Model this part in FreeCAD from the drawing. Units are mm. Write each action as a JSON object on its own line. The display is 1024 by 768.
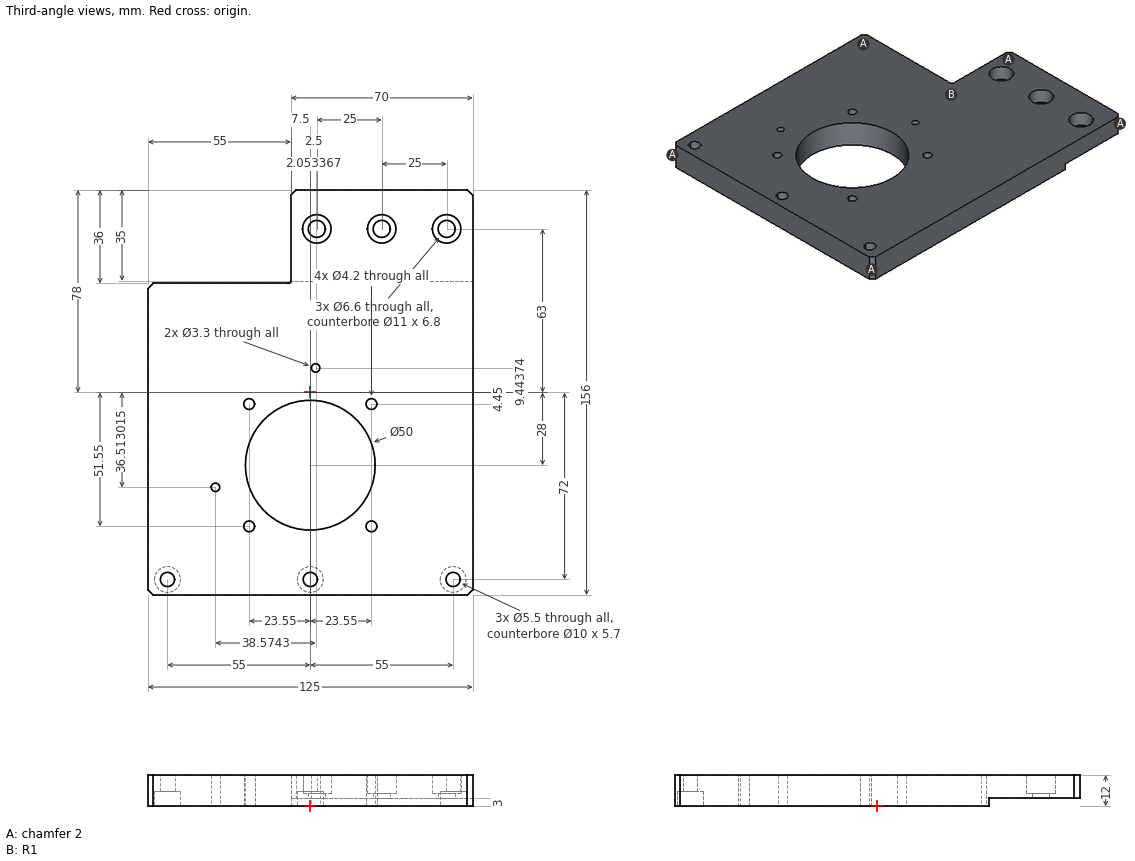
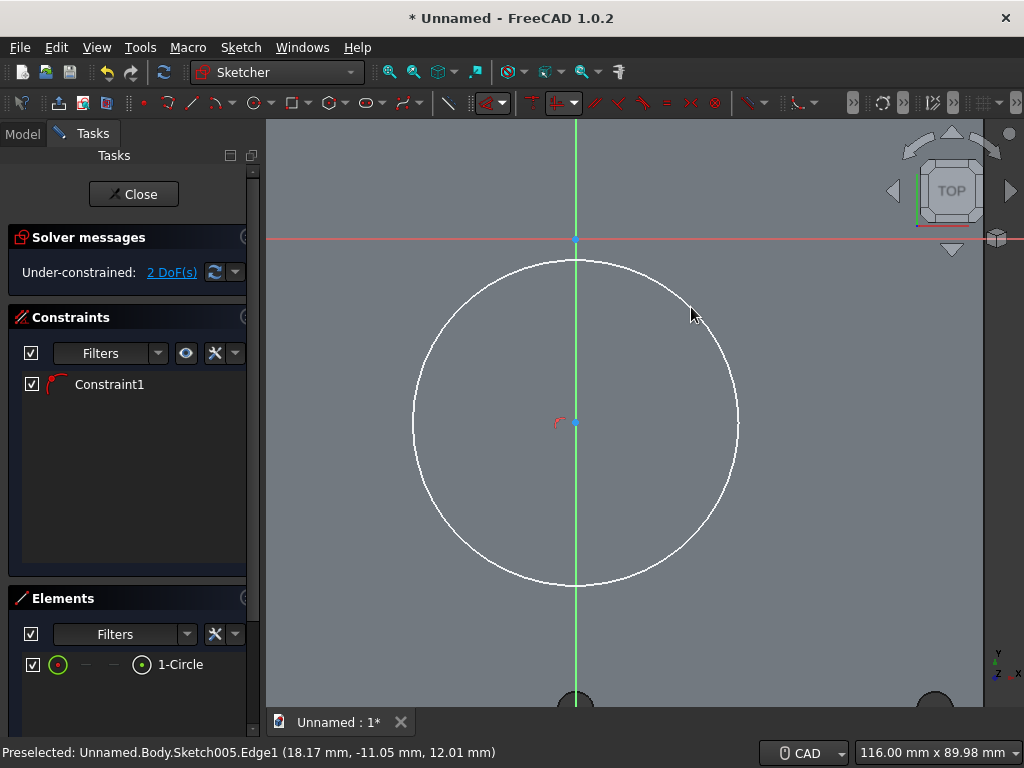
{"action": "left_click", "coordinate": [690, 307]}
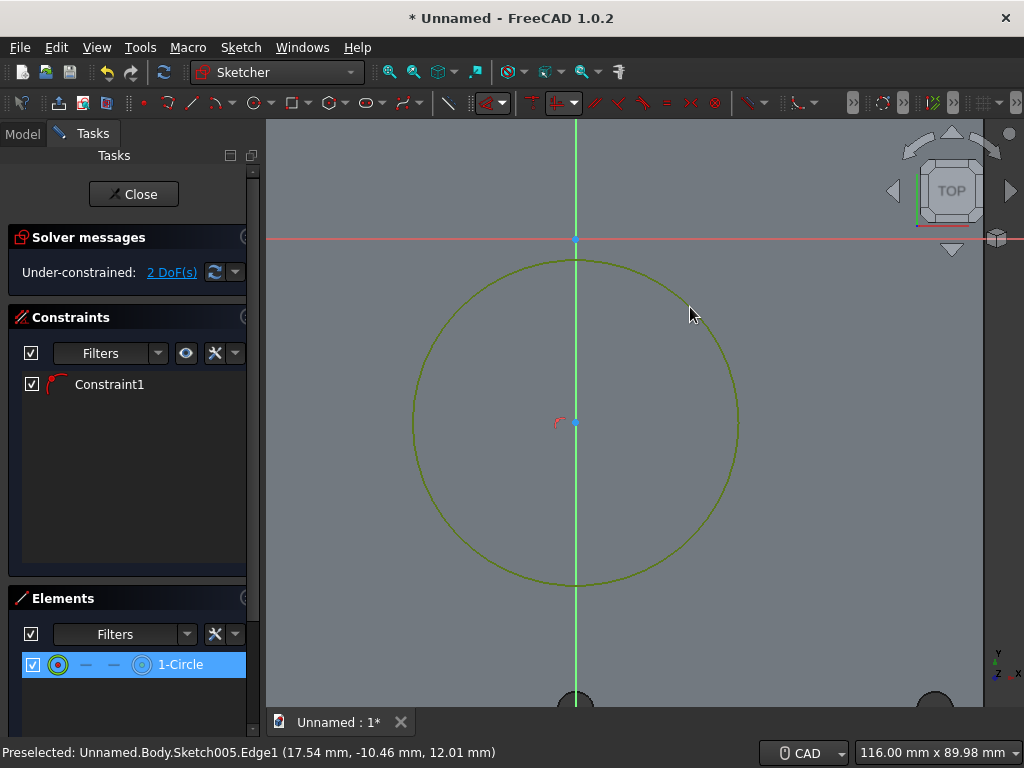
{"action": "left_click", "coordinate": [504, 104]}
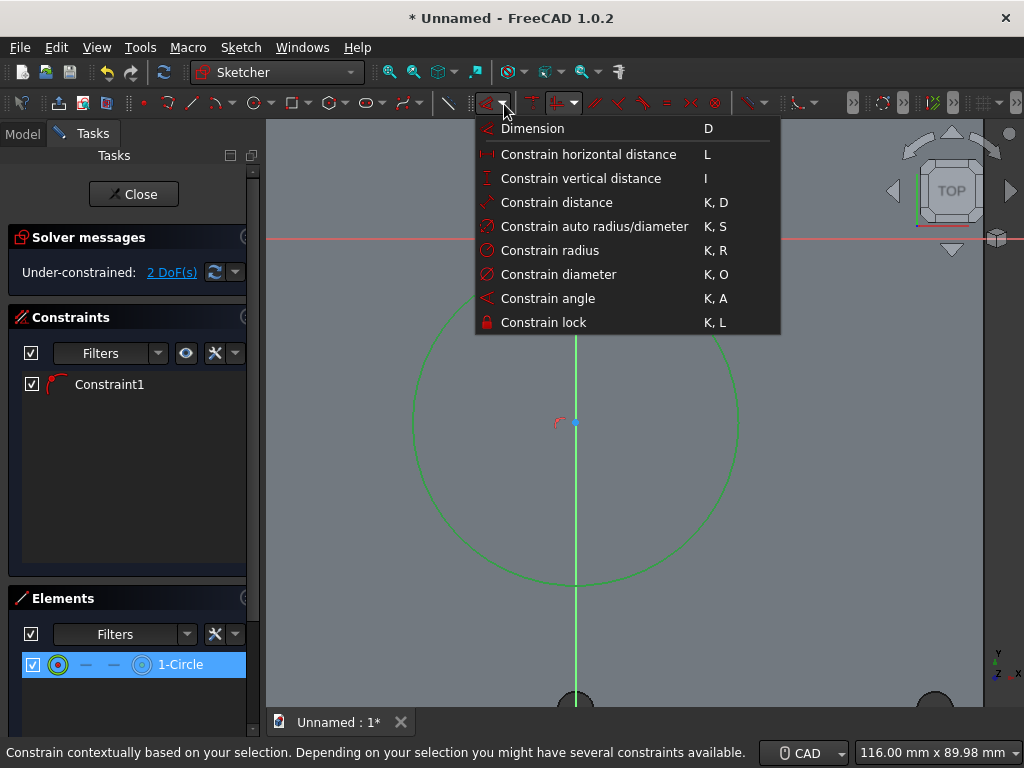
{"action": "left_click", "coordinate": [628, 274]}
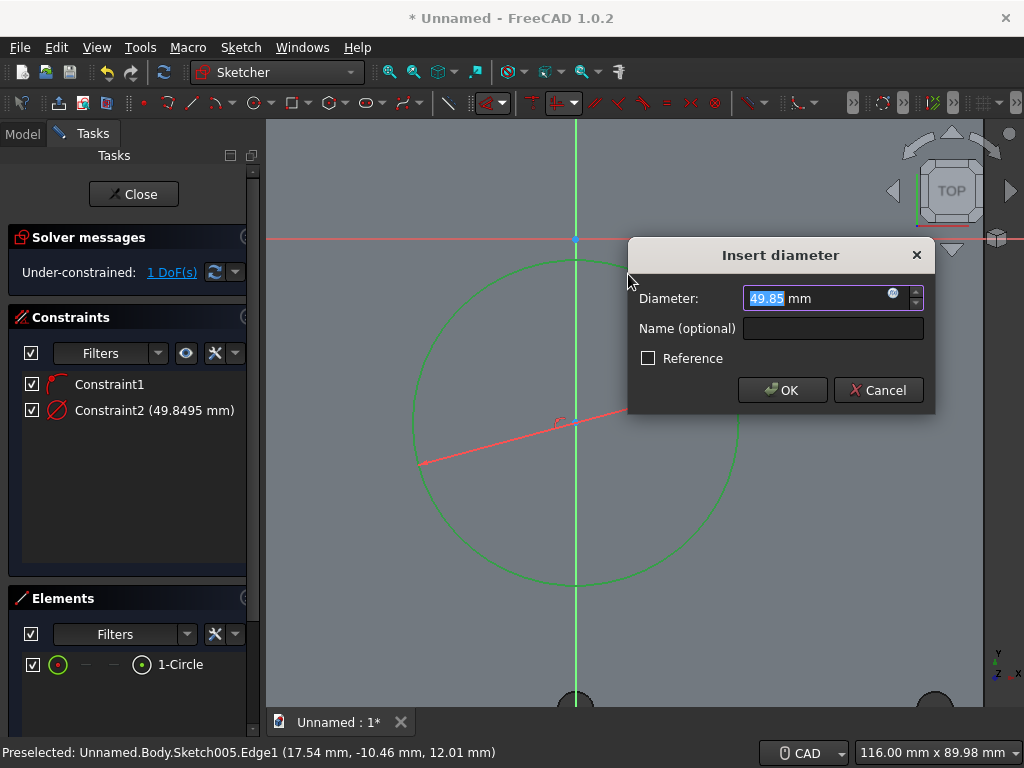
{"action": "type", "text": "50"}
{"action": "key", "text": "Return"}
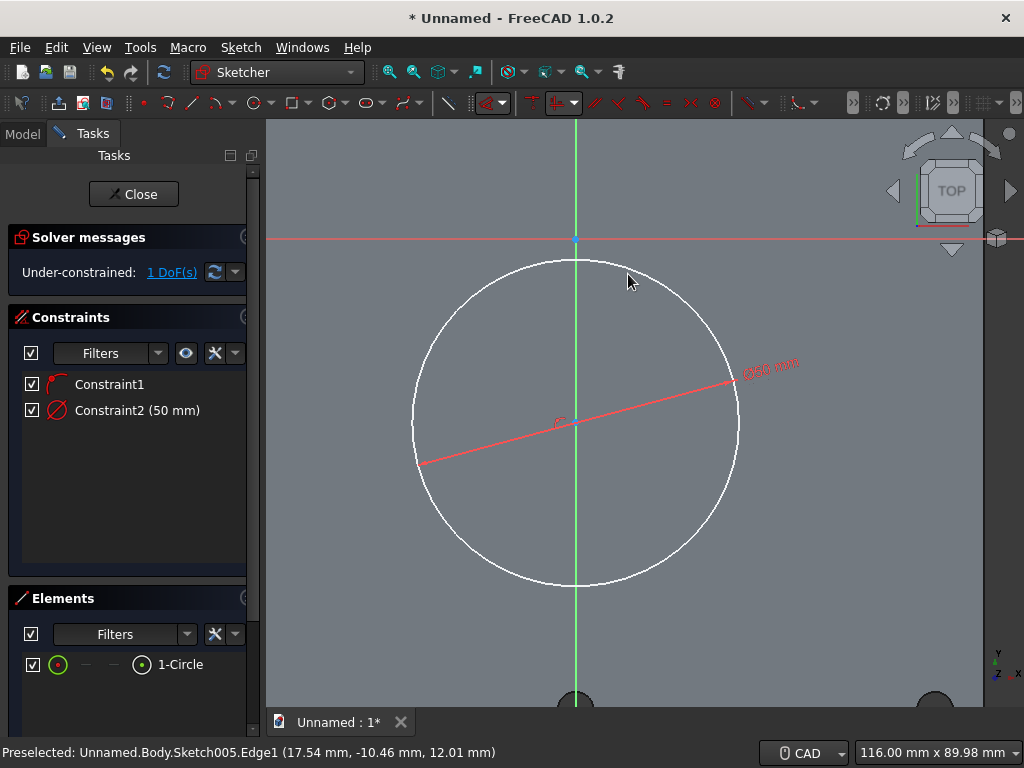
{"action": "left_click", "coordinate": [576, 423]}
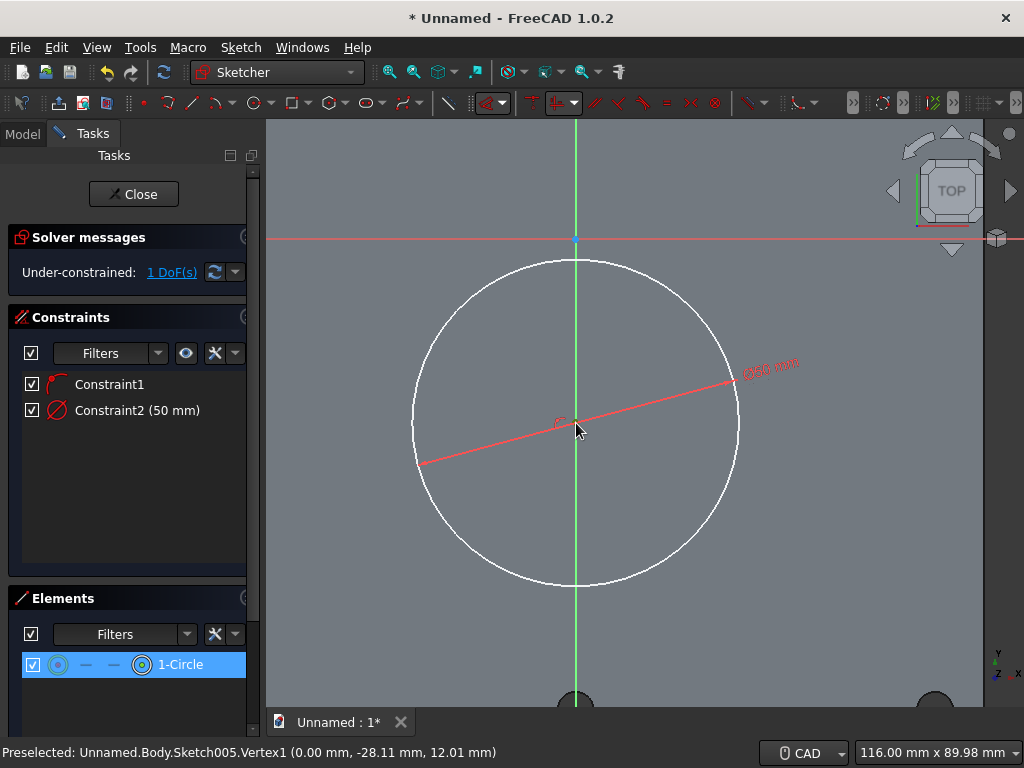
{"action": "left_click", "coordinate": [504, 104]}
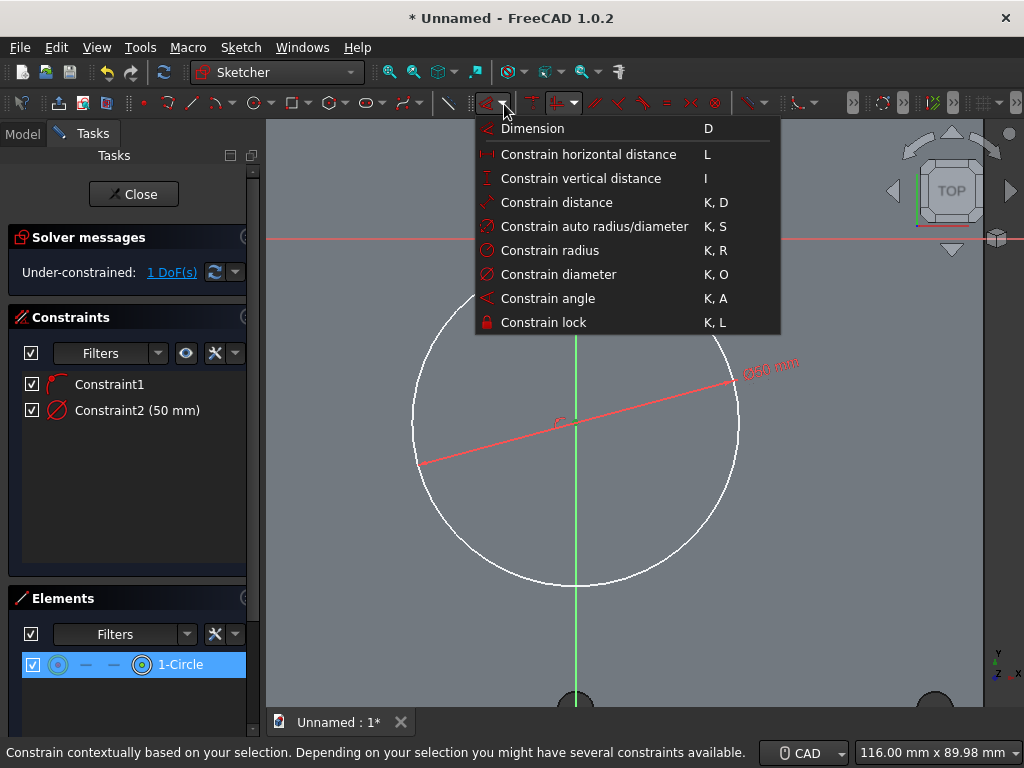
{"action": "left_click", "coordinate": [628, 178]}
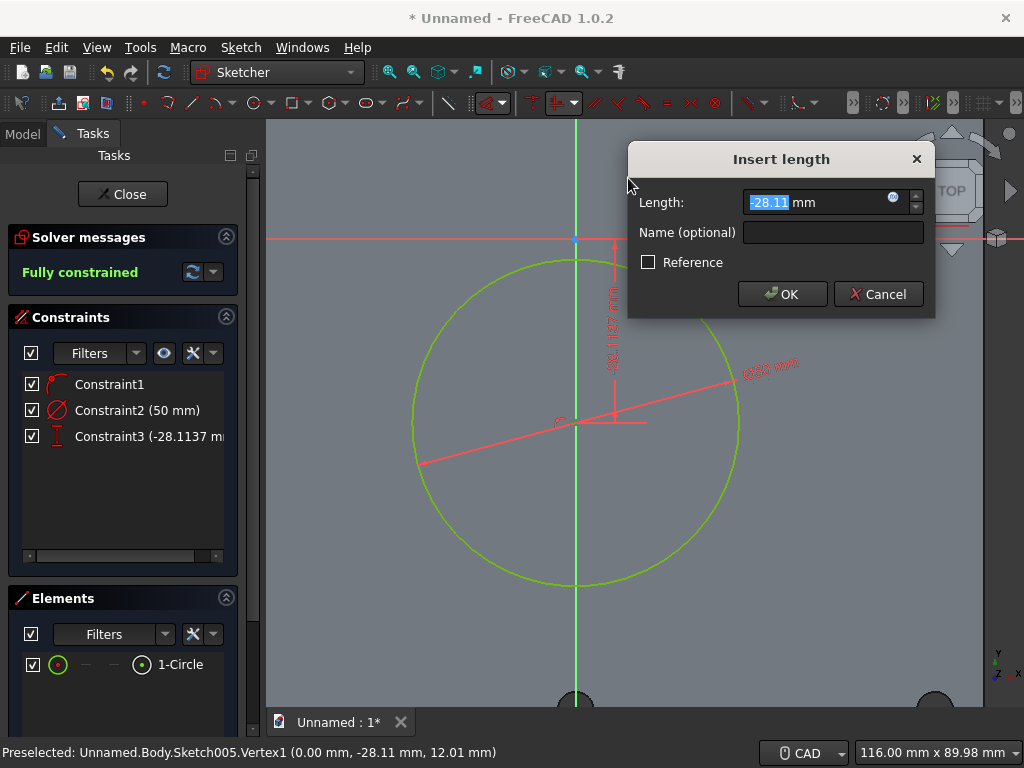
{"action": "type", "text": "-28"}
{"action": "key", "text": "Return"}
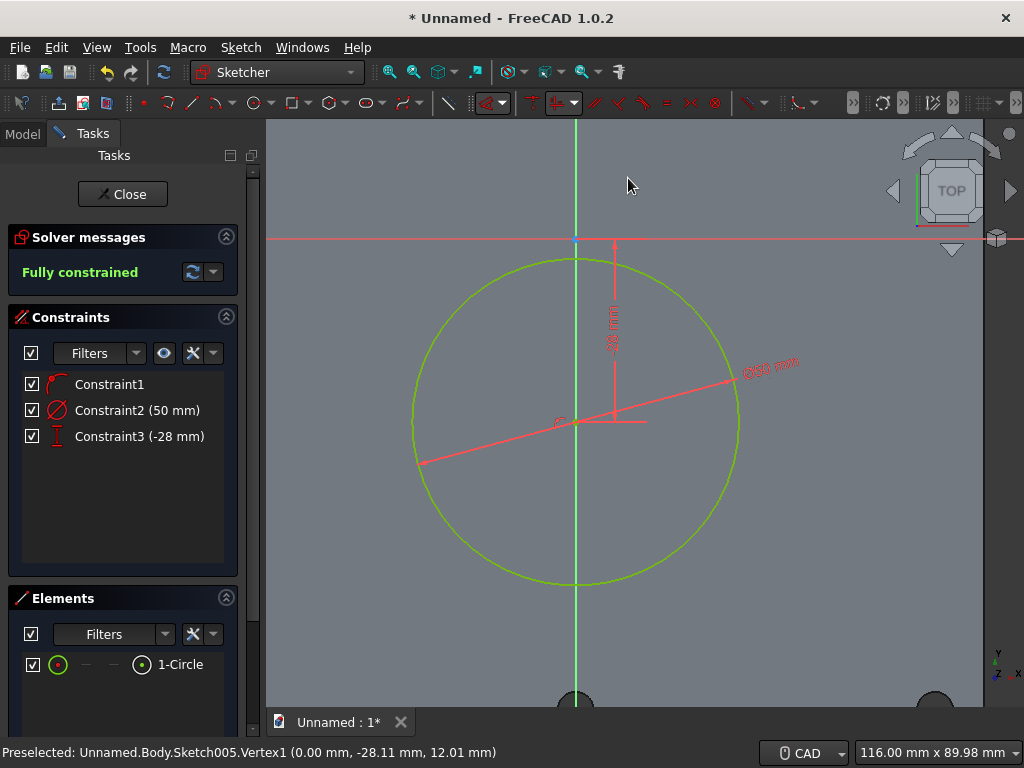
{"action": "left_click", "coordinate": [123, 194]}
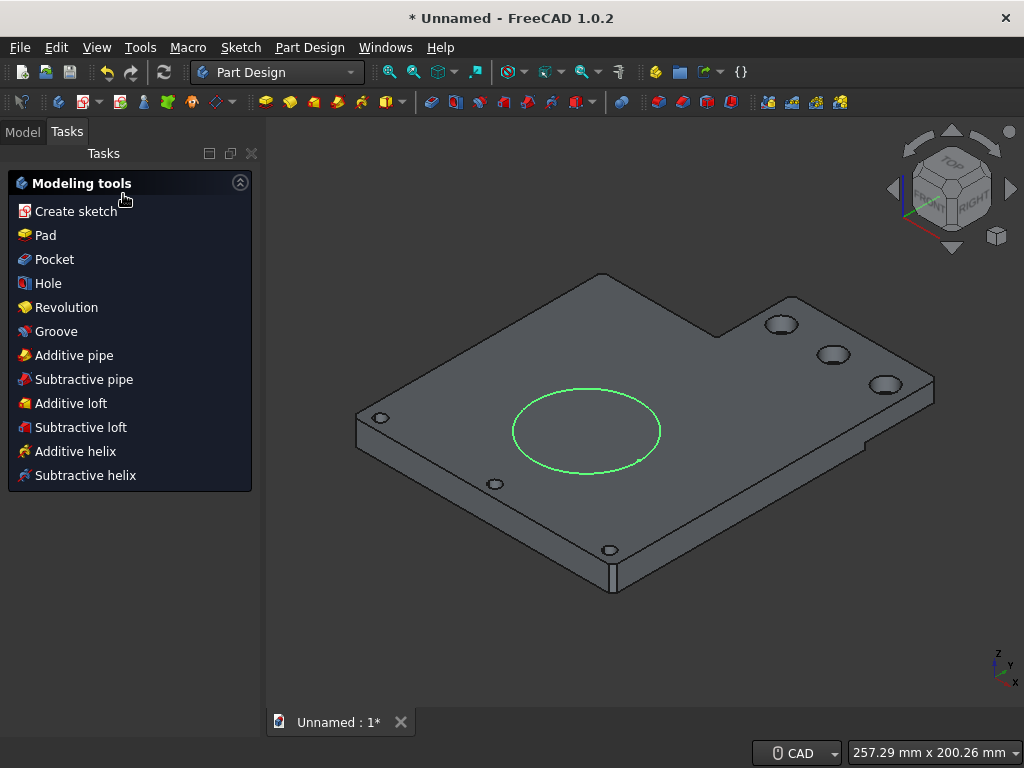
{"action": "left_click", "coordinate": [432, 102]}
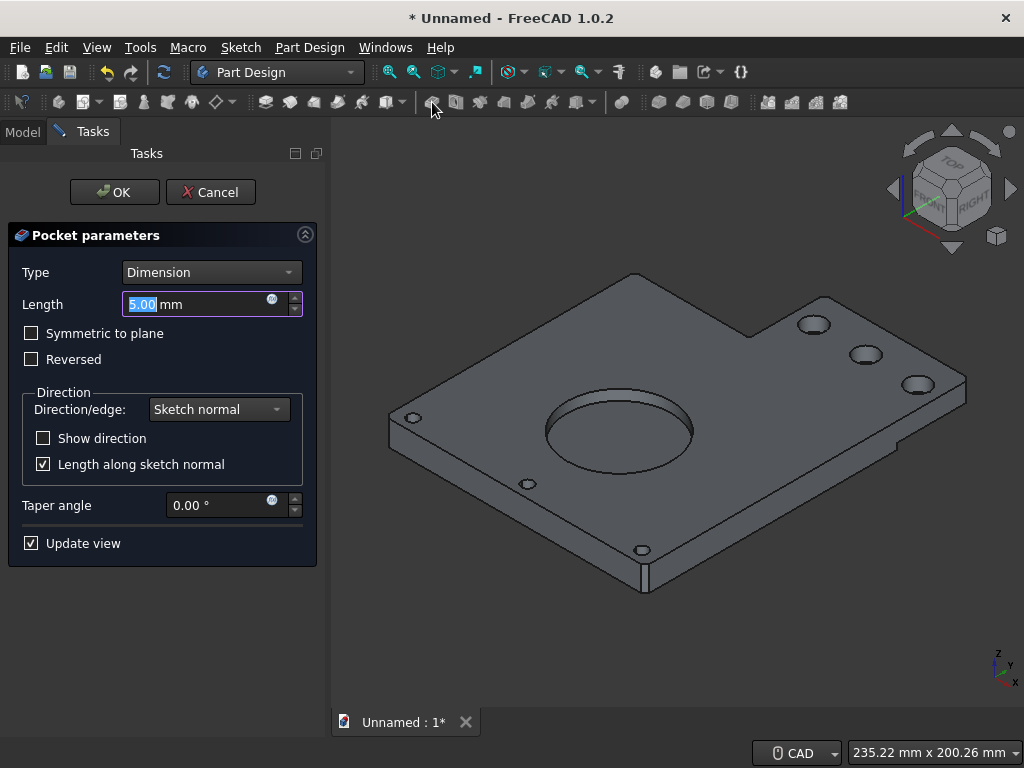
{"action": "left_click", "coordinate": [212, 272]}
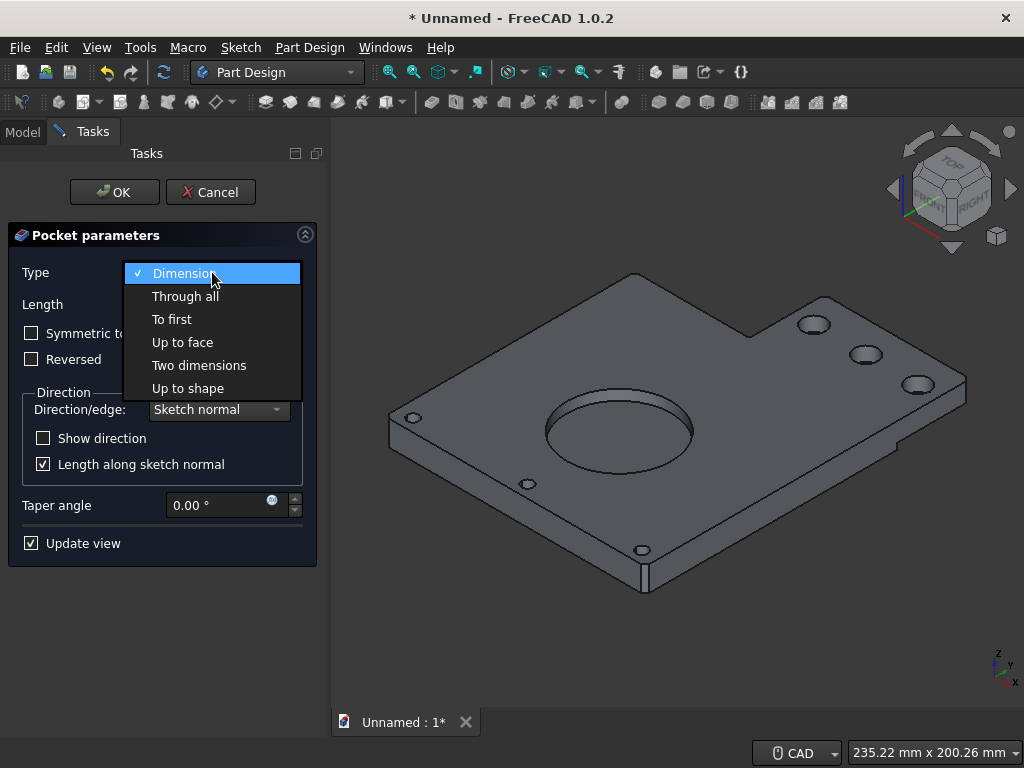
{"action": "left_click", "coordinate": [212, 296]}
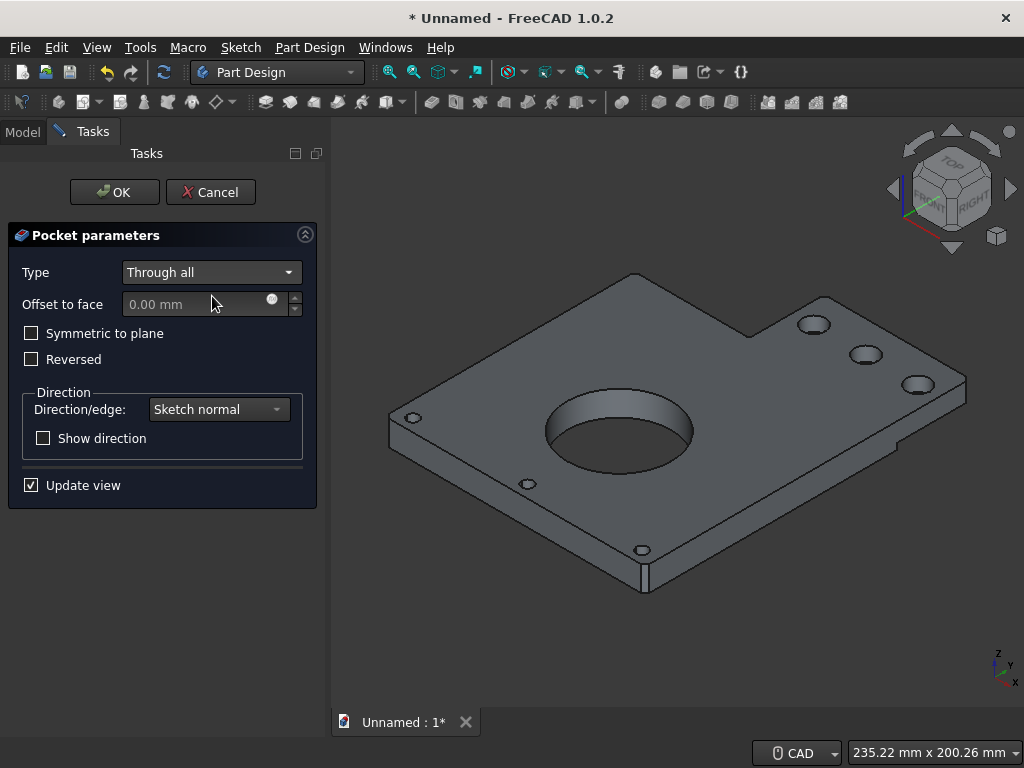
{"action": "left_click", "coordinate": [115, 192]}